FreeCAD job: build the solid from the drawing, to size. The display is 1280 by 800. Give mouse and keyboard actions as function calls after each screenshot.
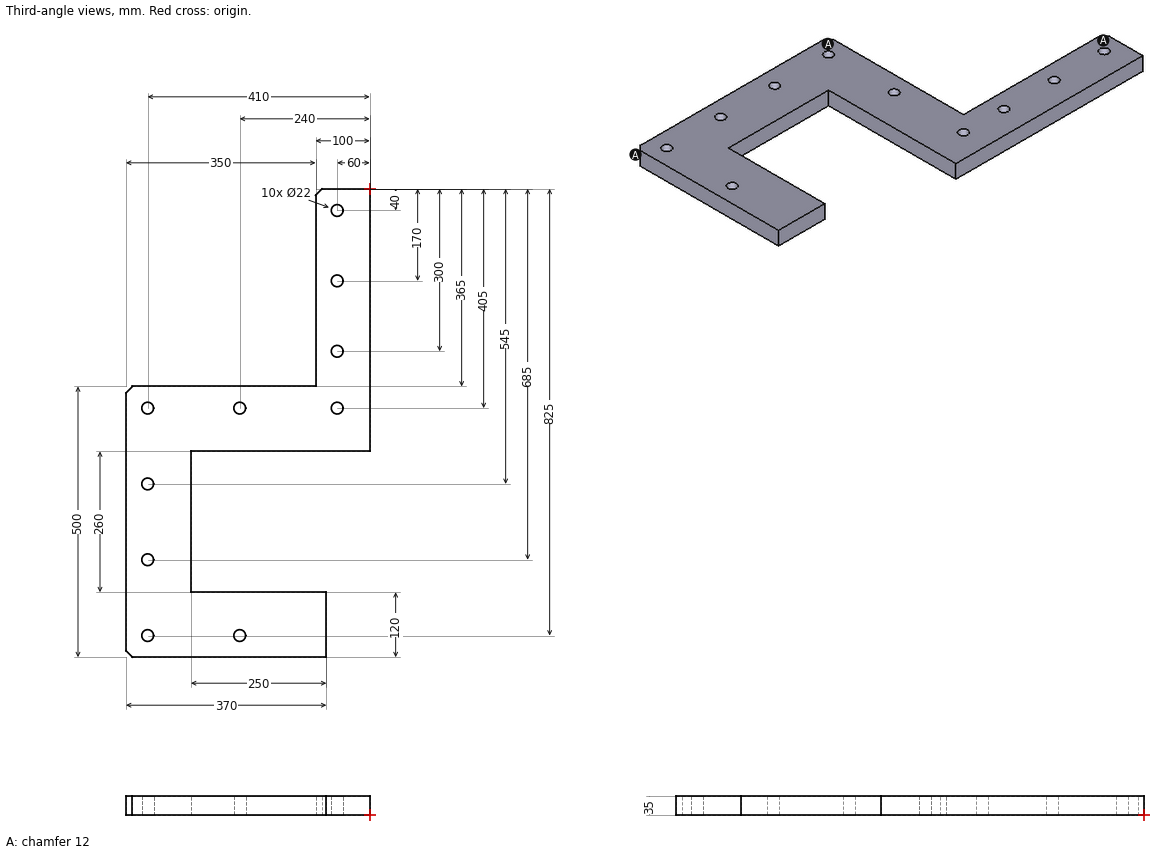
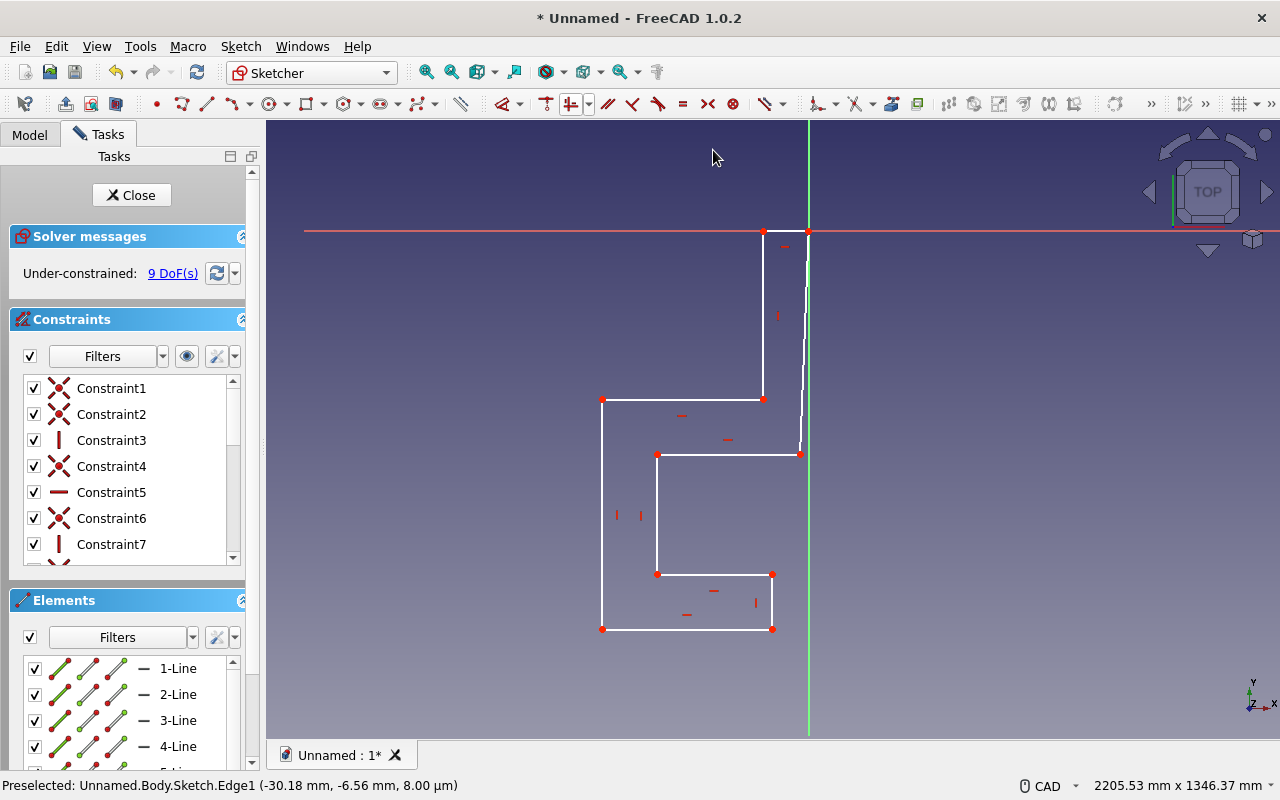
click(806, 298)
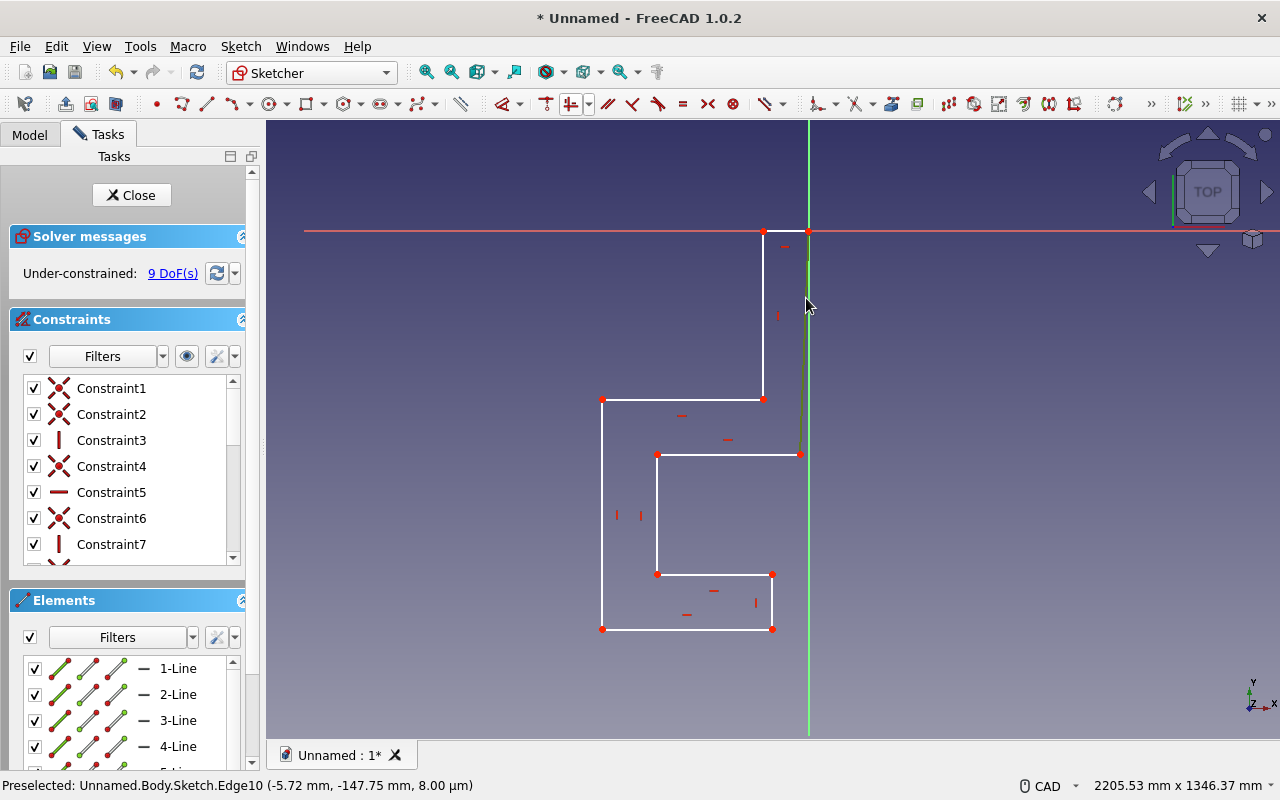
click(588, 104)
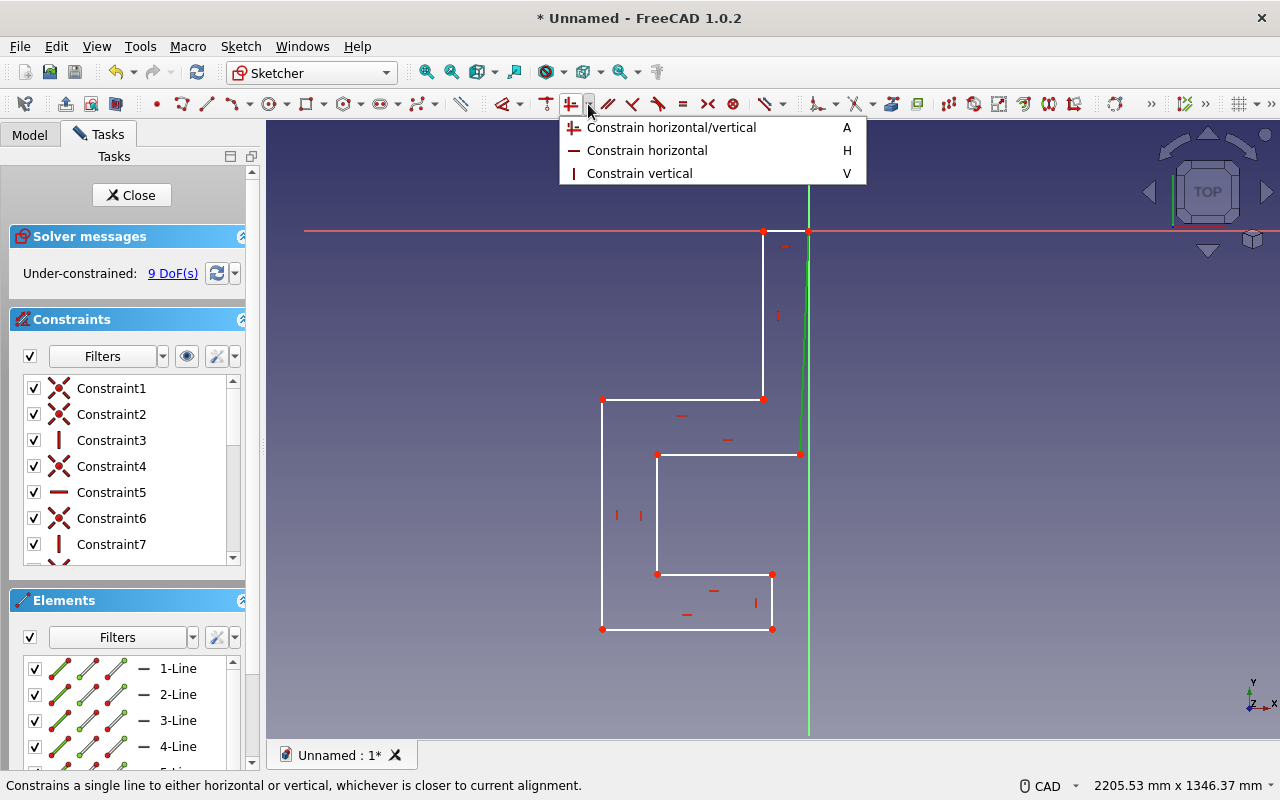
click(713, 174)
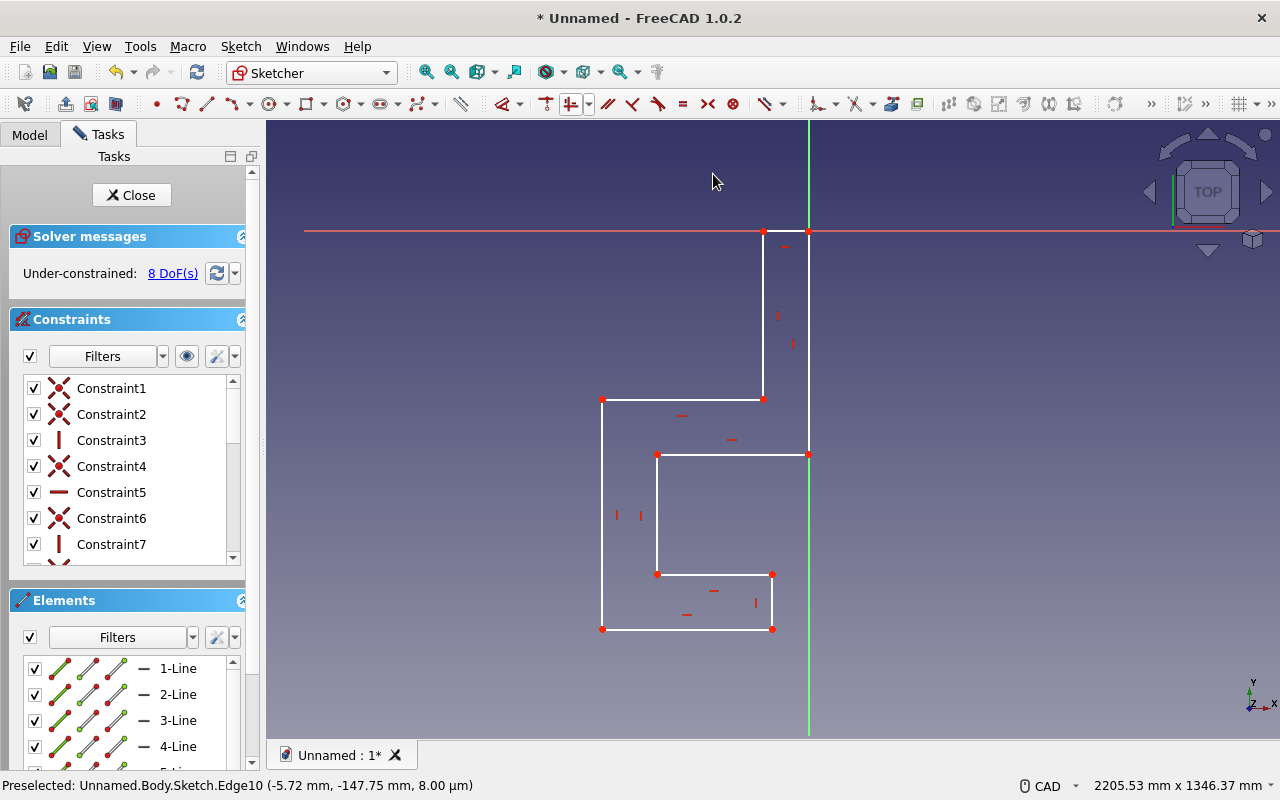
click(795, 231)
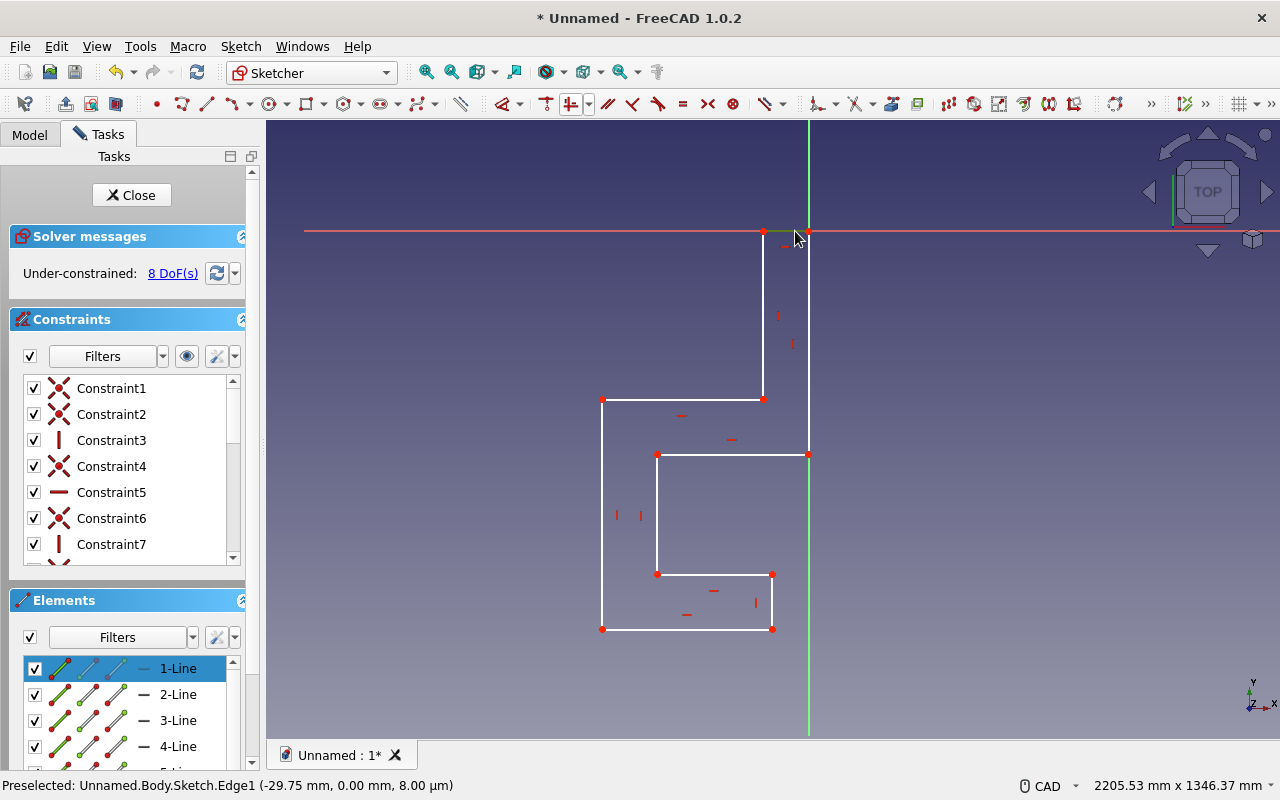
click(520, 104)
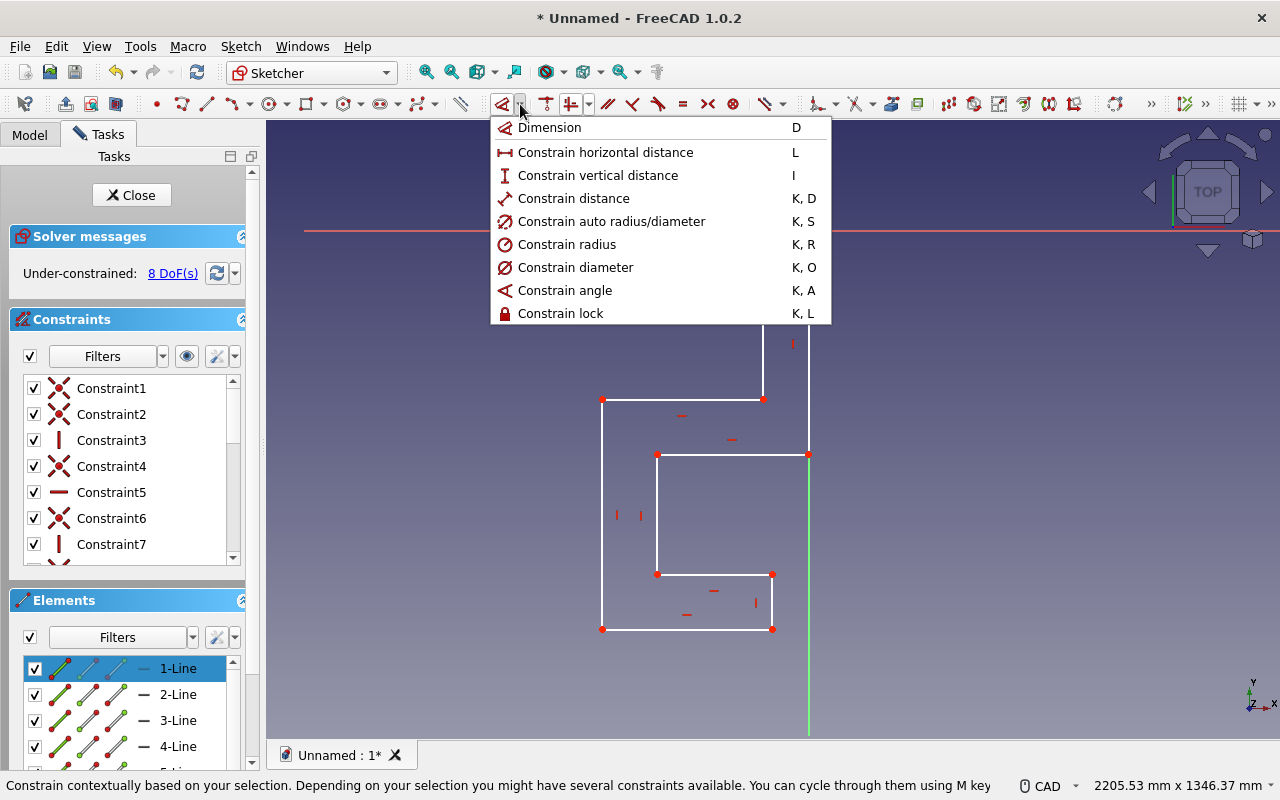
click(661, 152)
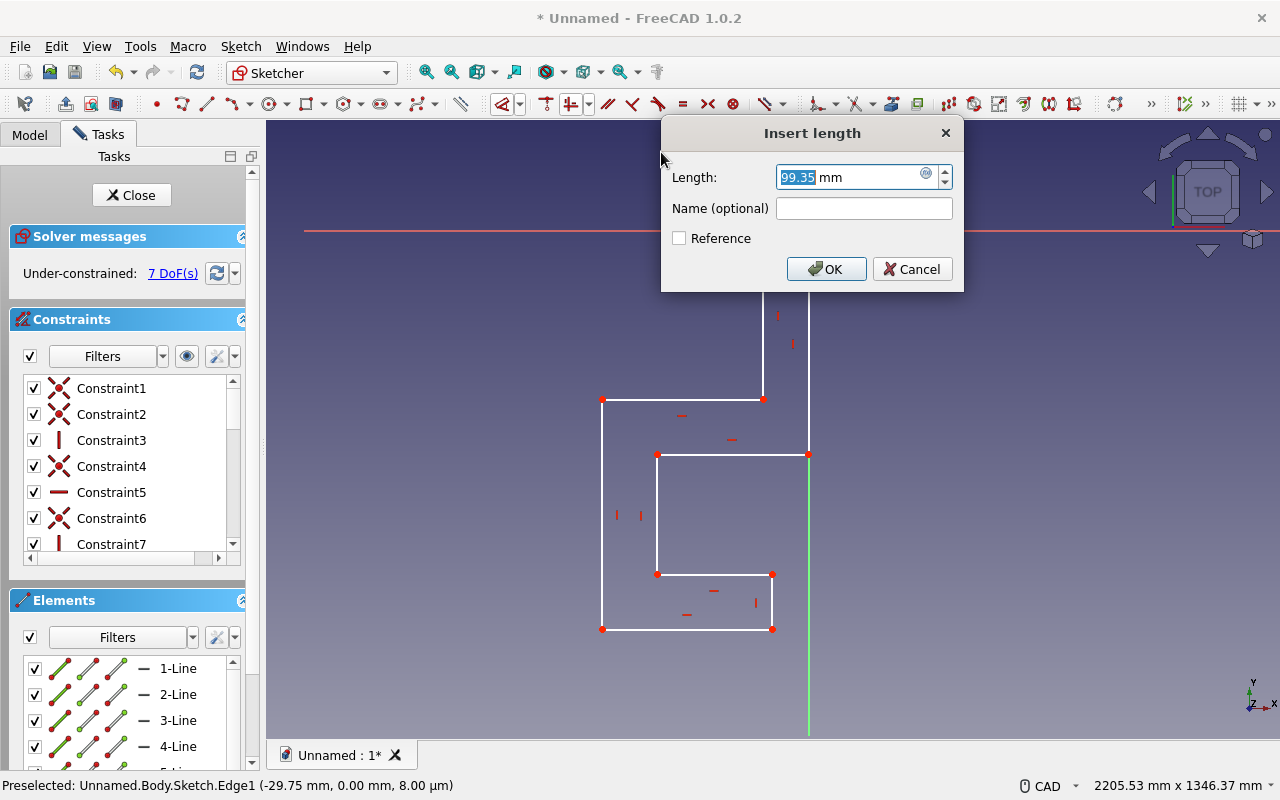
text(100)
key(Return)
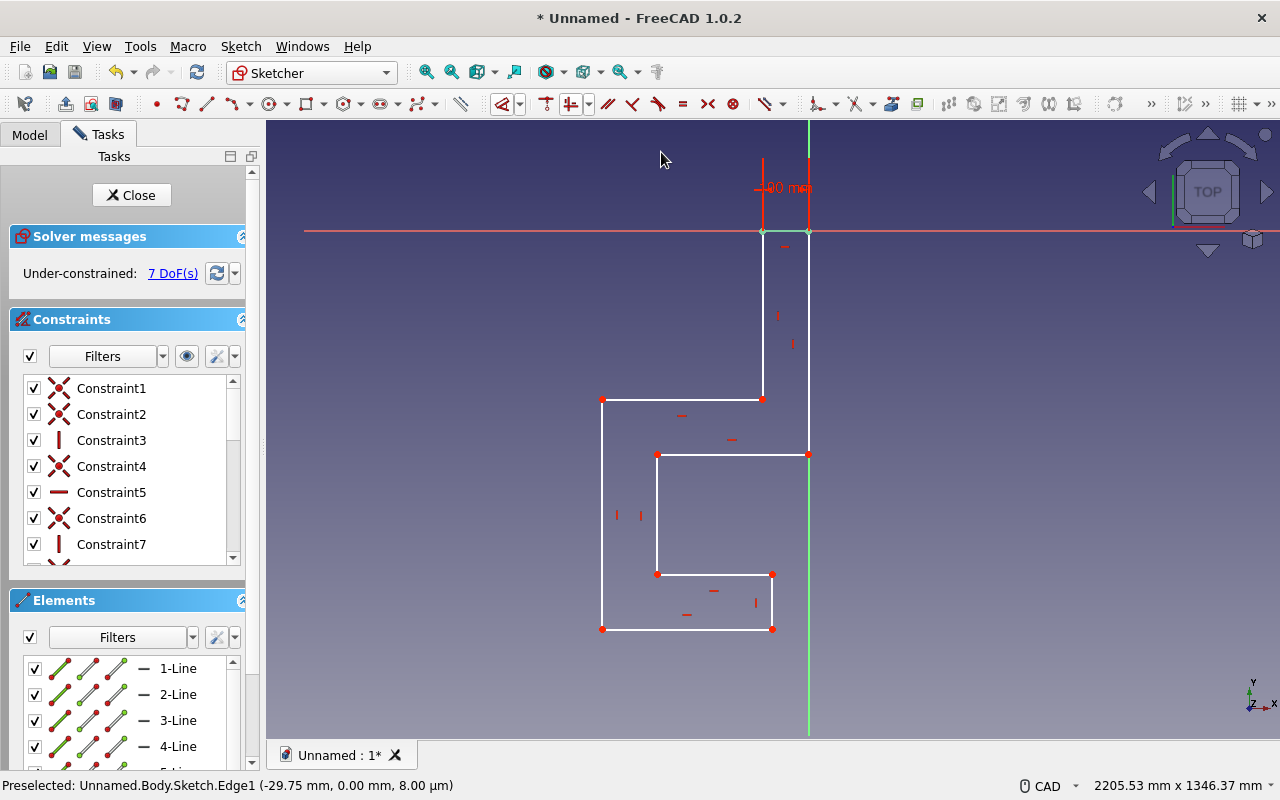
click(763, 282)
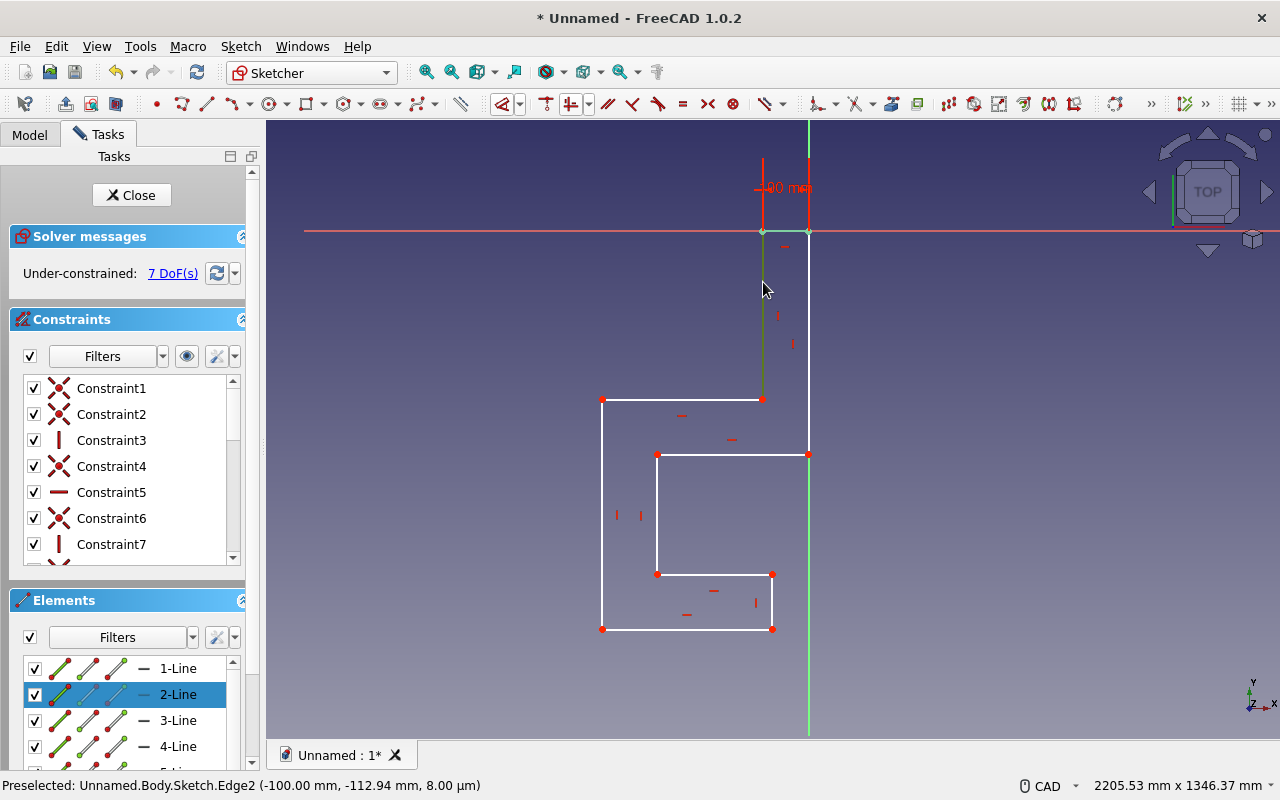
click(520, 104)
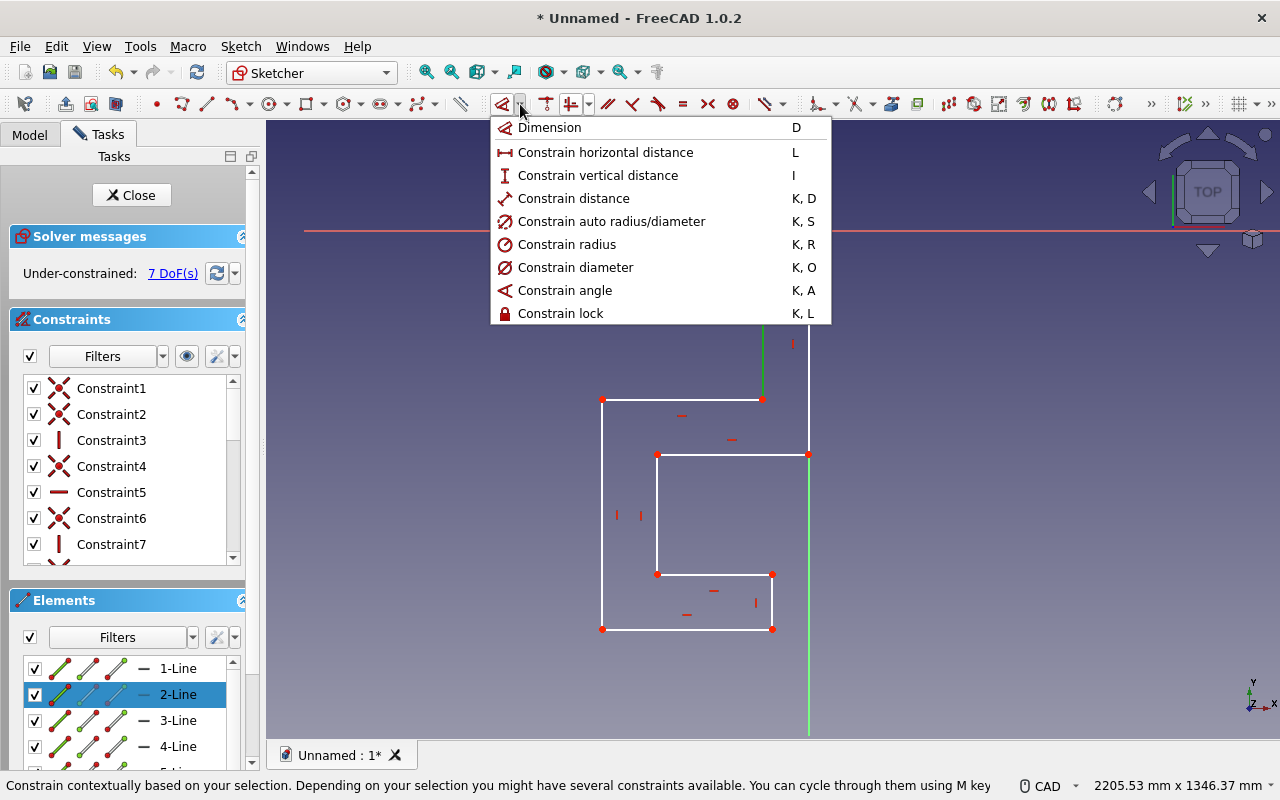
click(661, 176)